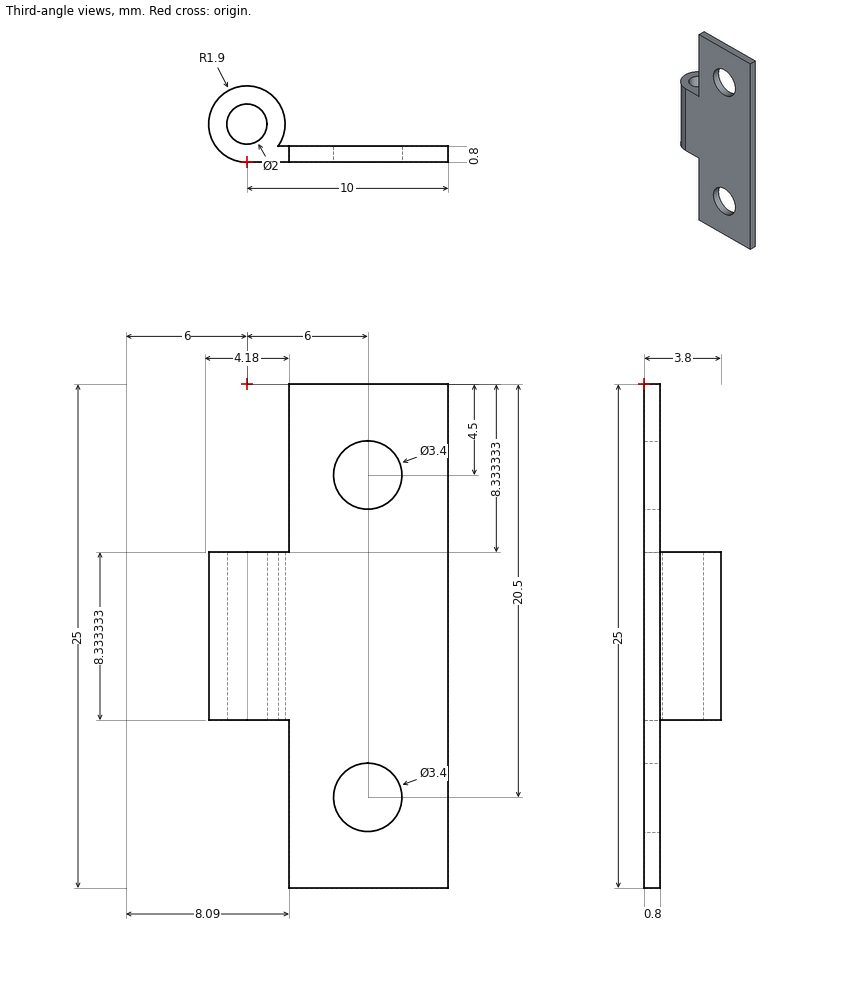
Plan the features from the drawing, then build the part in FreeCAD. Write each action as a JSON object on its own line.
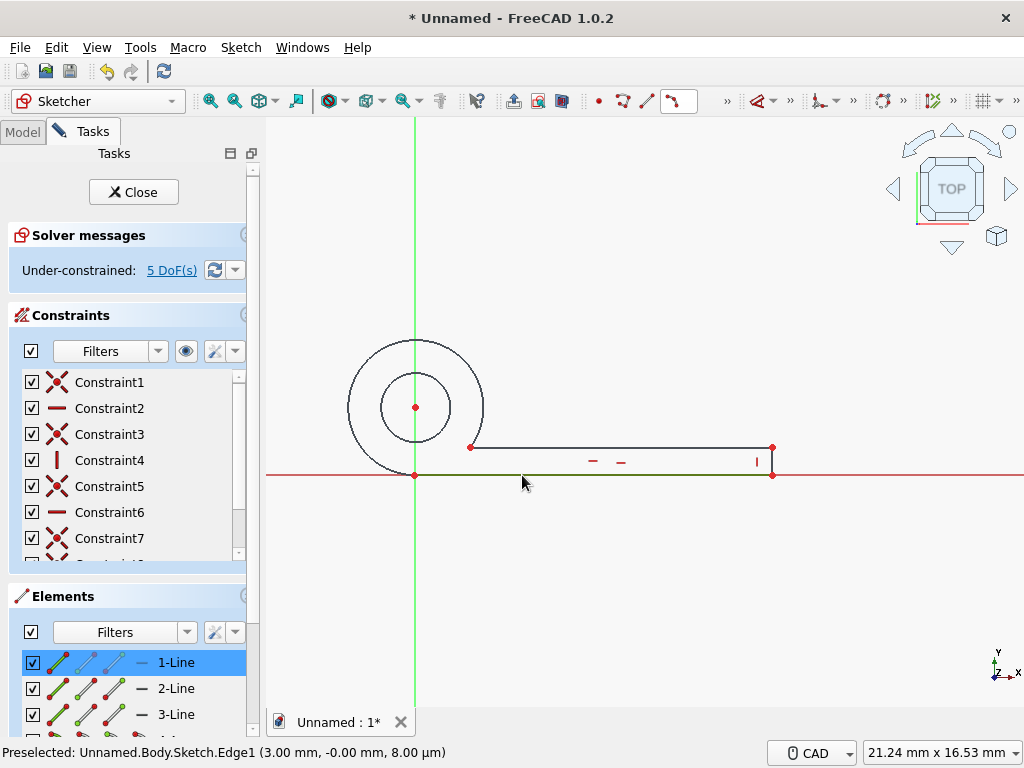
{"action": "left_click", "coordinate": [454, 352]}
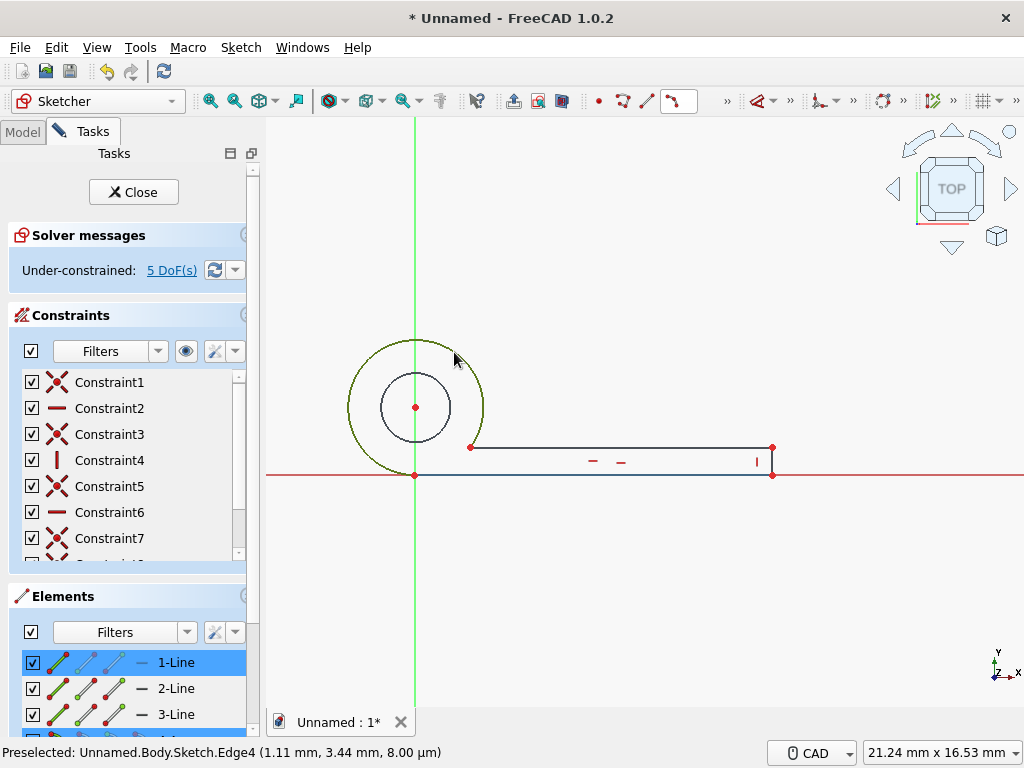
{"action": "key", "text": "t"}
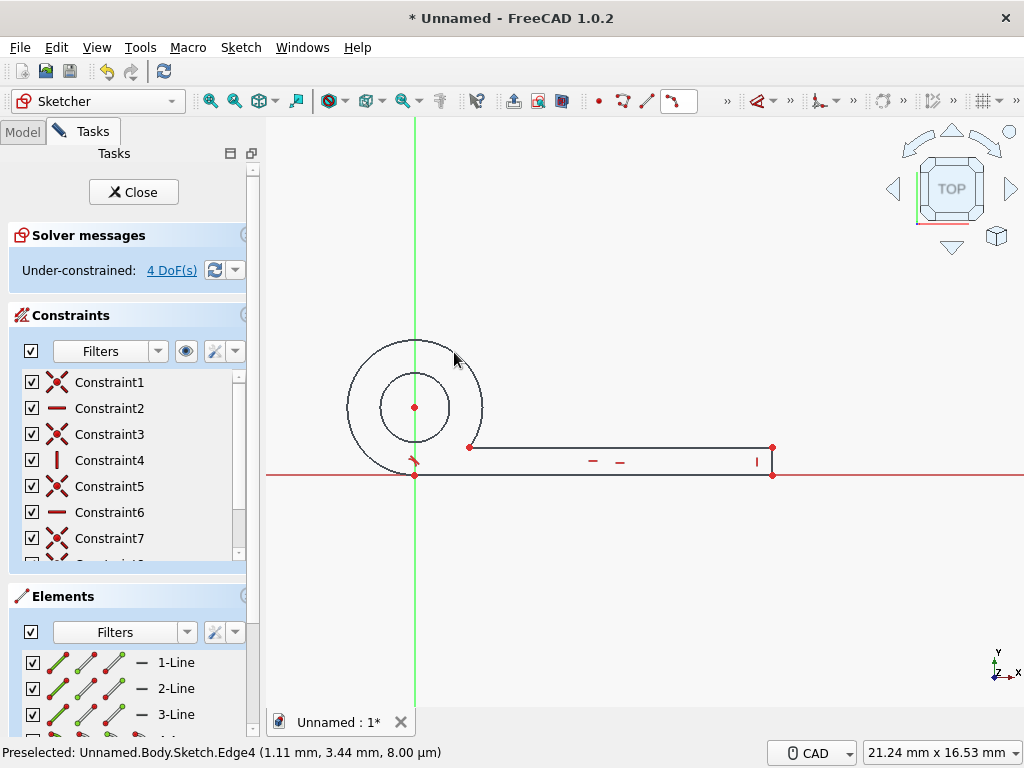
{"action": "left_click", "coordinate": [758, 102]}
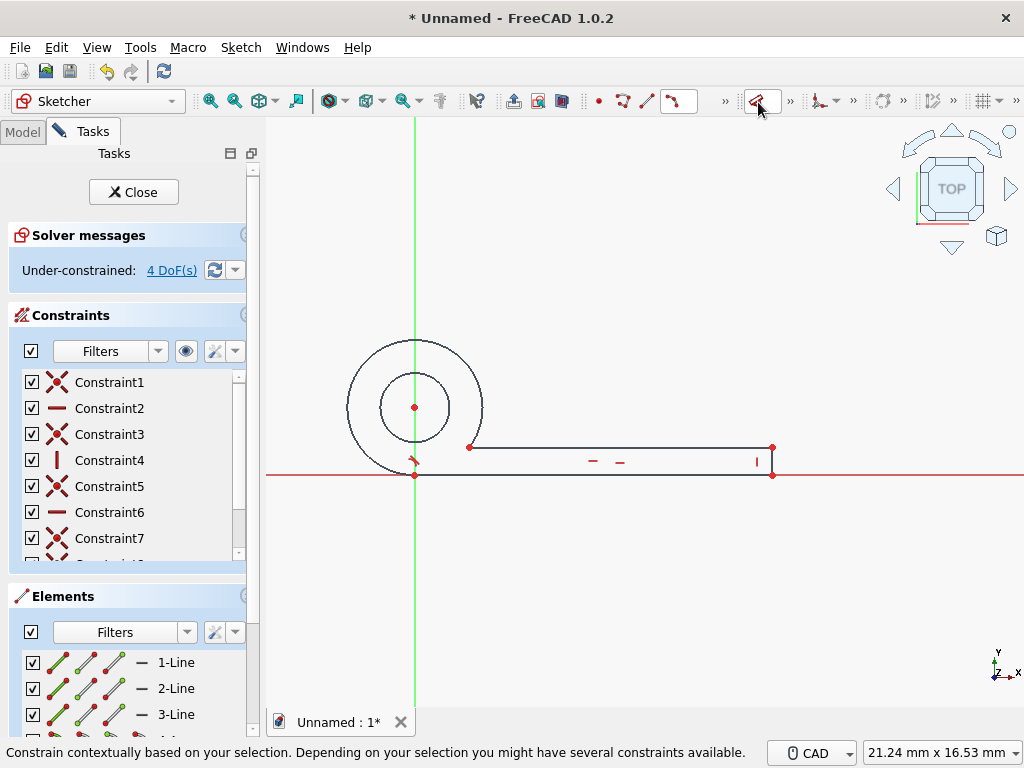
{"action": "left_click", "coordinate": [453, 352]}
{"action": "left_click", "coordinate": [471, 326]}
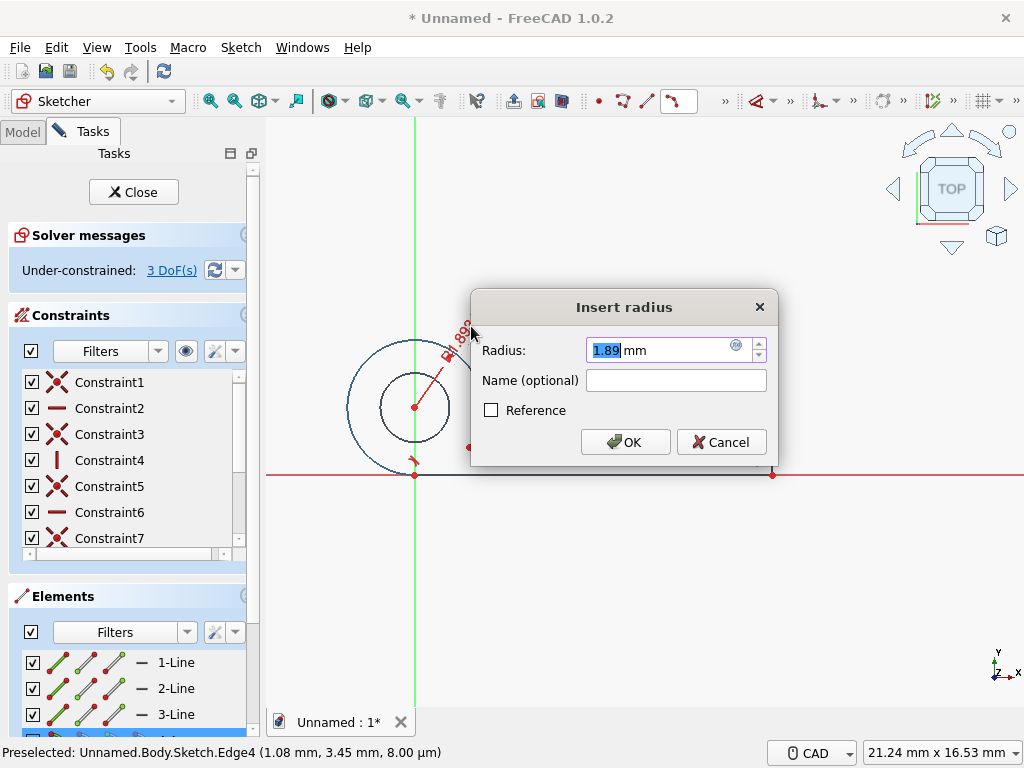
{"action": "type", "text": "1.9"}
{"action": "key", "text": "Return"}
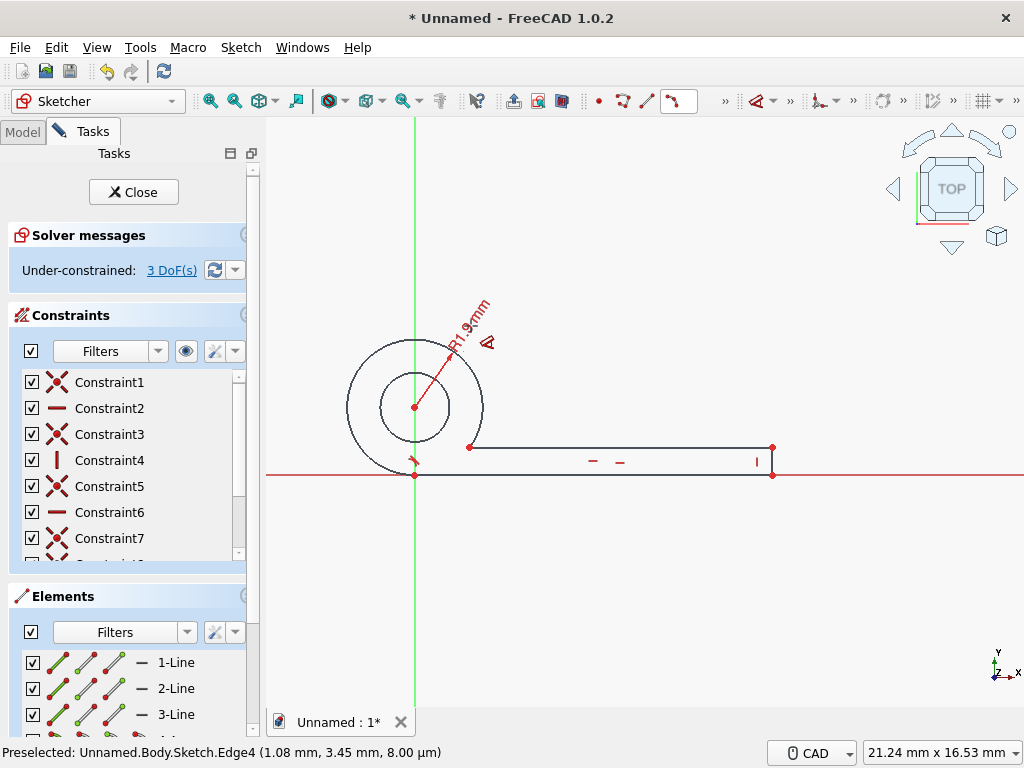
{"action": "left_click", "coordinate": [439, 383]}
{"action": "left_click", "coordinate": [500, 382]}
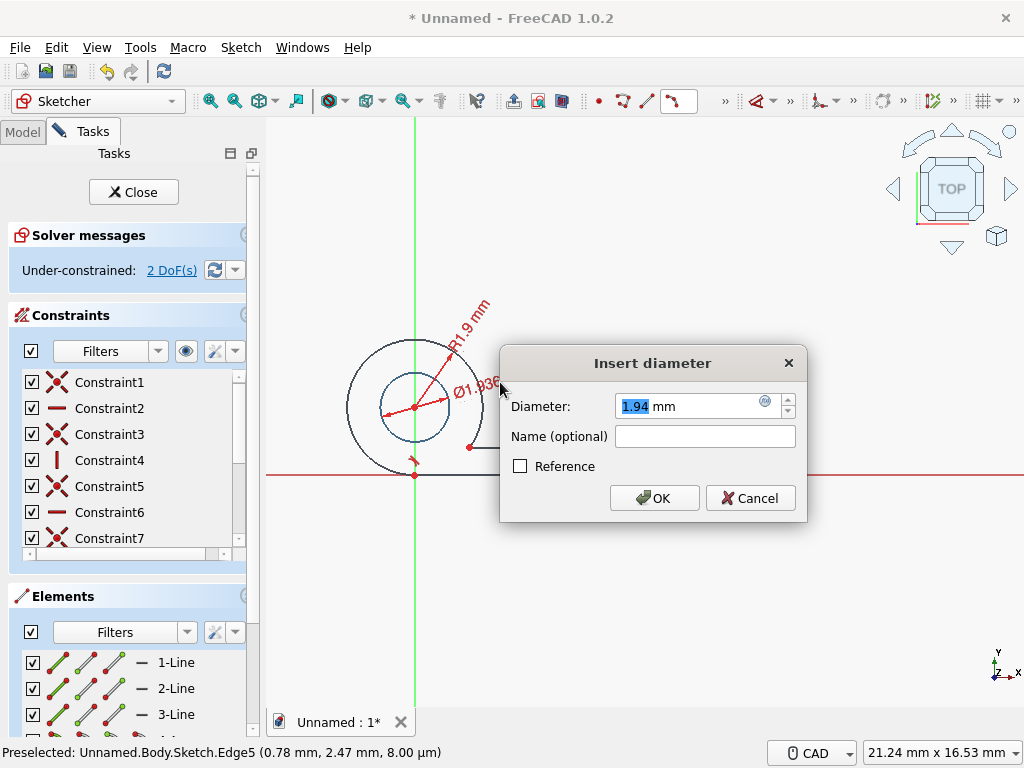
{"action": "type", "text": "2"}
{"action": "key", "text": "Return"}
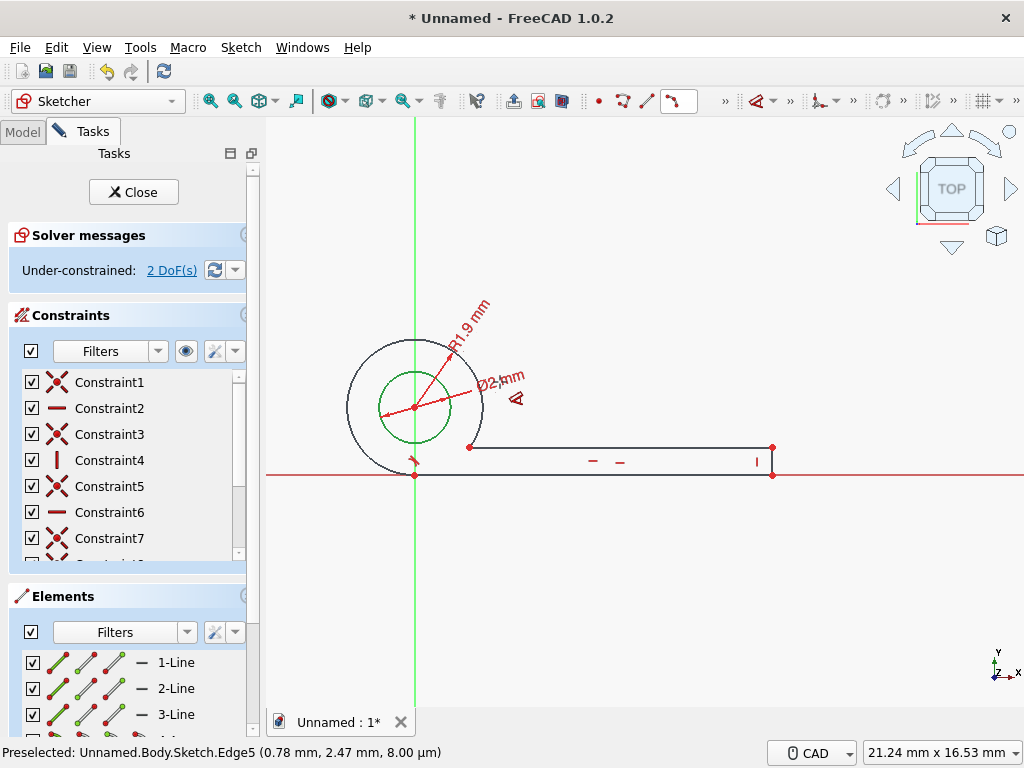
{"action": "left_click", "coordinate": [522, 475]}
{"action": "left_click", "coordinate": [593, 509]}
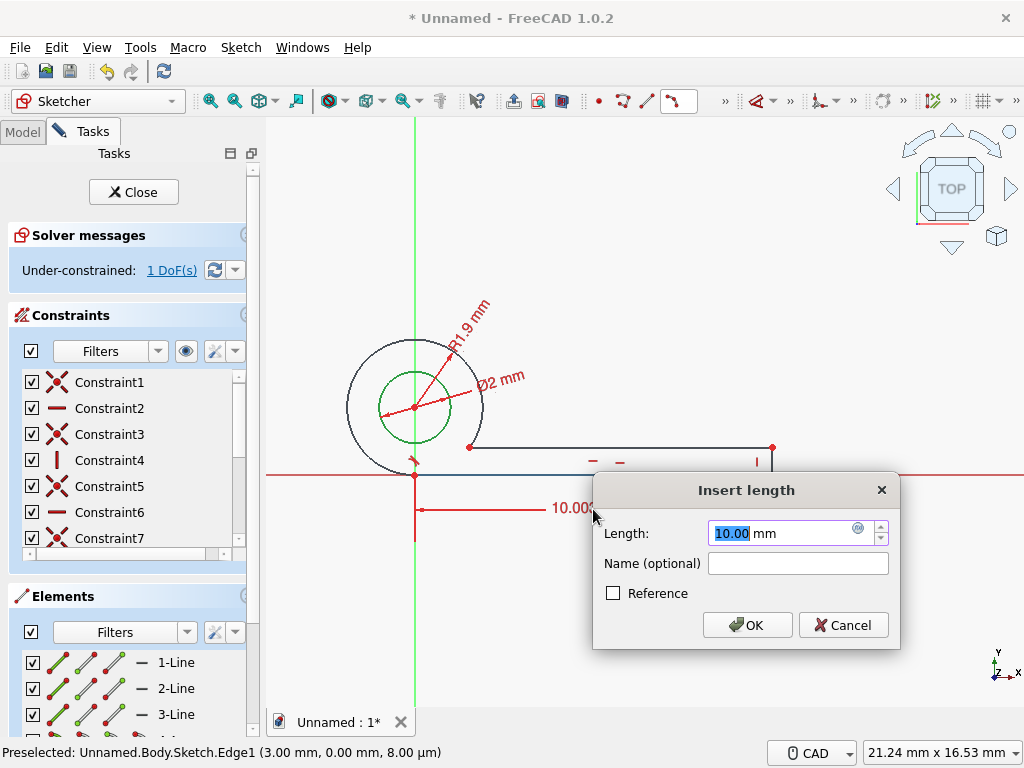
{"action": "type", "text": "10"}
{"action": "key", "text": "Return"}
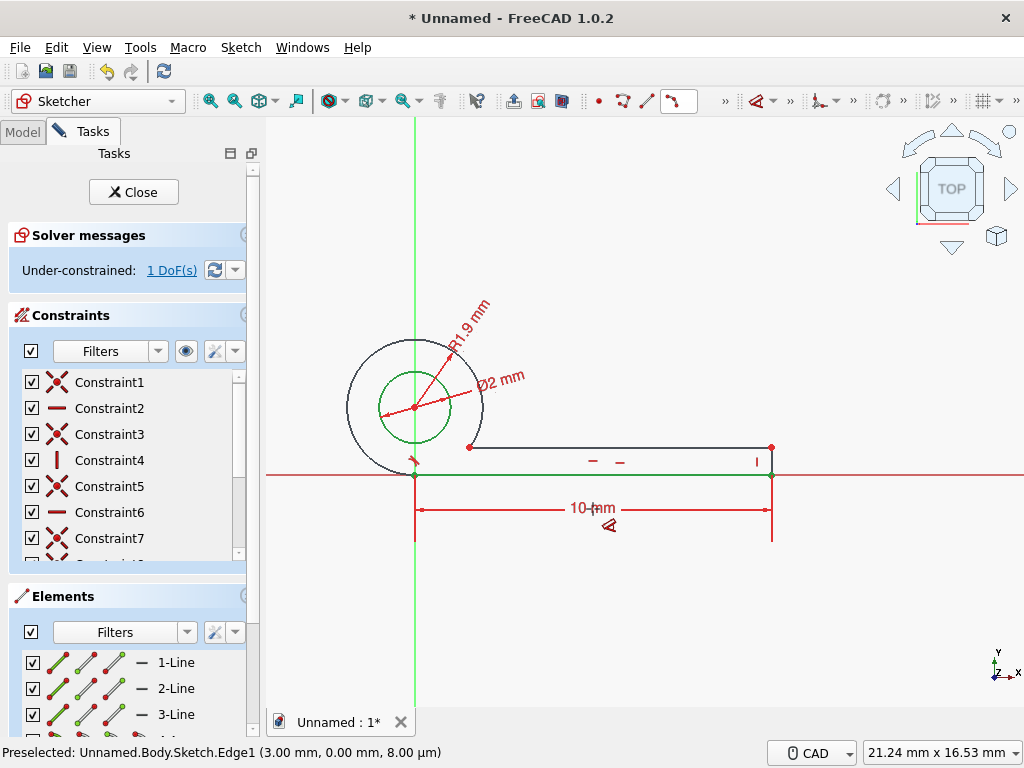
{"action": "scroll", "coordinate": [772, 464], "scroll_direction": "up", "scroll_amount": 2}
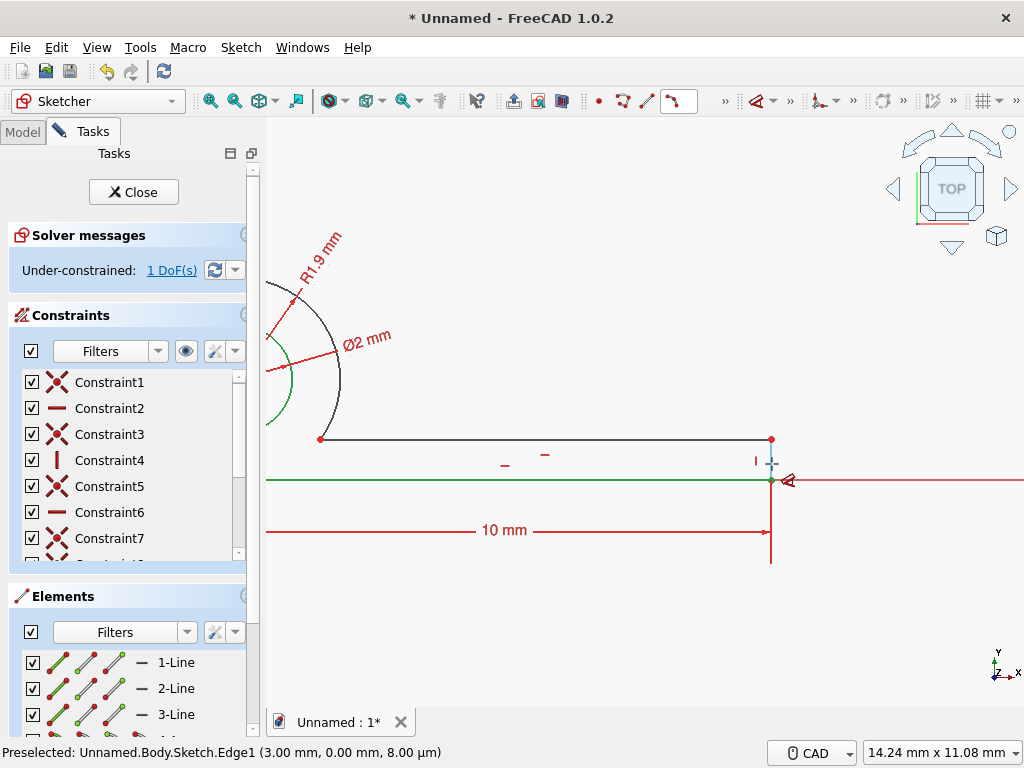
{"action": "left_click", "coordinate": [771, 464]}
{"action": "left_click", "coordinate": [805, 460]}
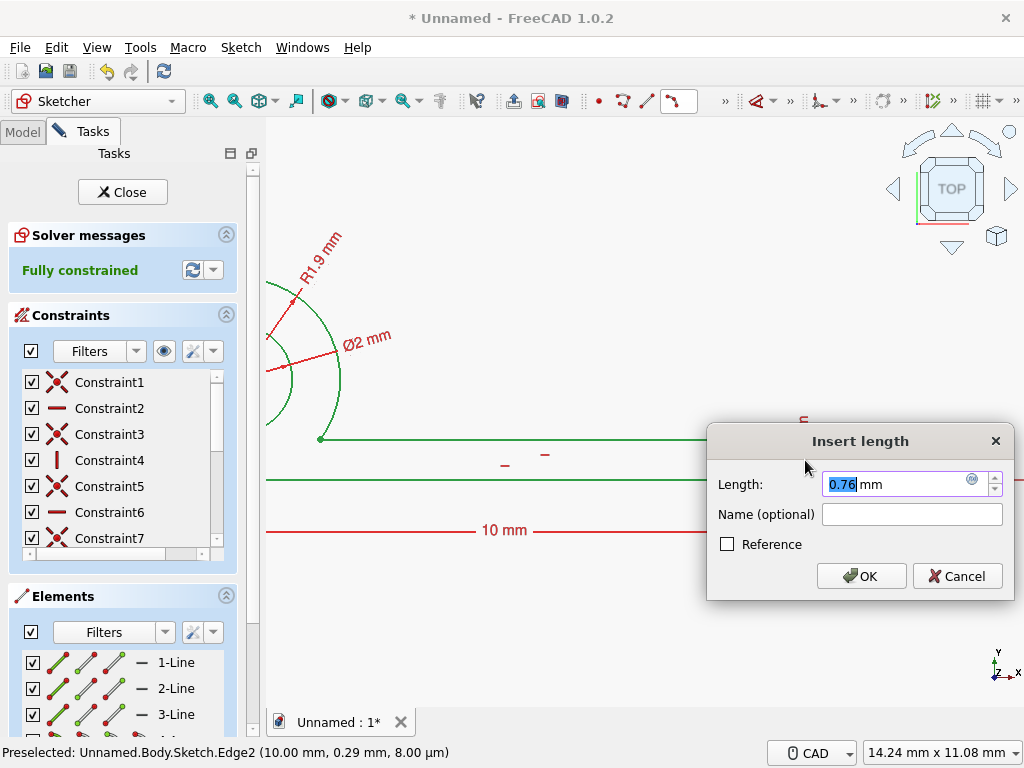
{"action": "type", "text": "0.8"}
{"action": "key", "text": "Return"}
{"action": "key", "text": "Escape"}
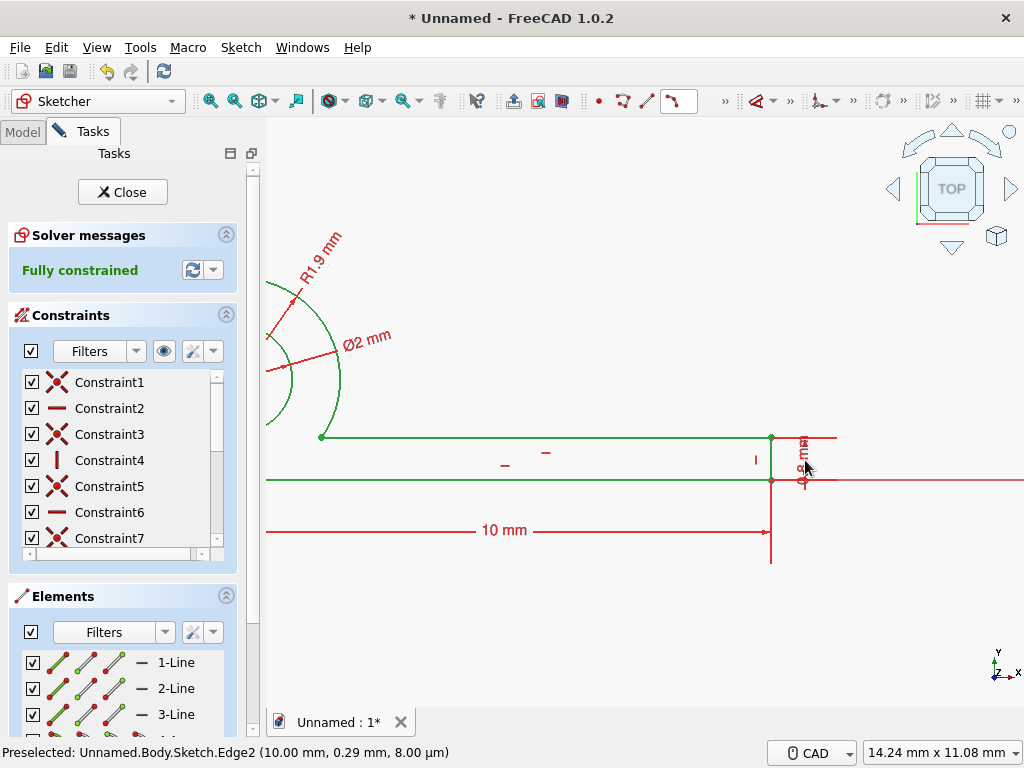
{"action": "left_click", "coordinate": [123, 192]}